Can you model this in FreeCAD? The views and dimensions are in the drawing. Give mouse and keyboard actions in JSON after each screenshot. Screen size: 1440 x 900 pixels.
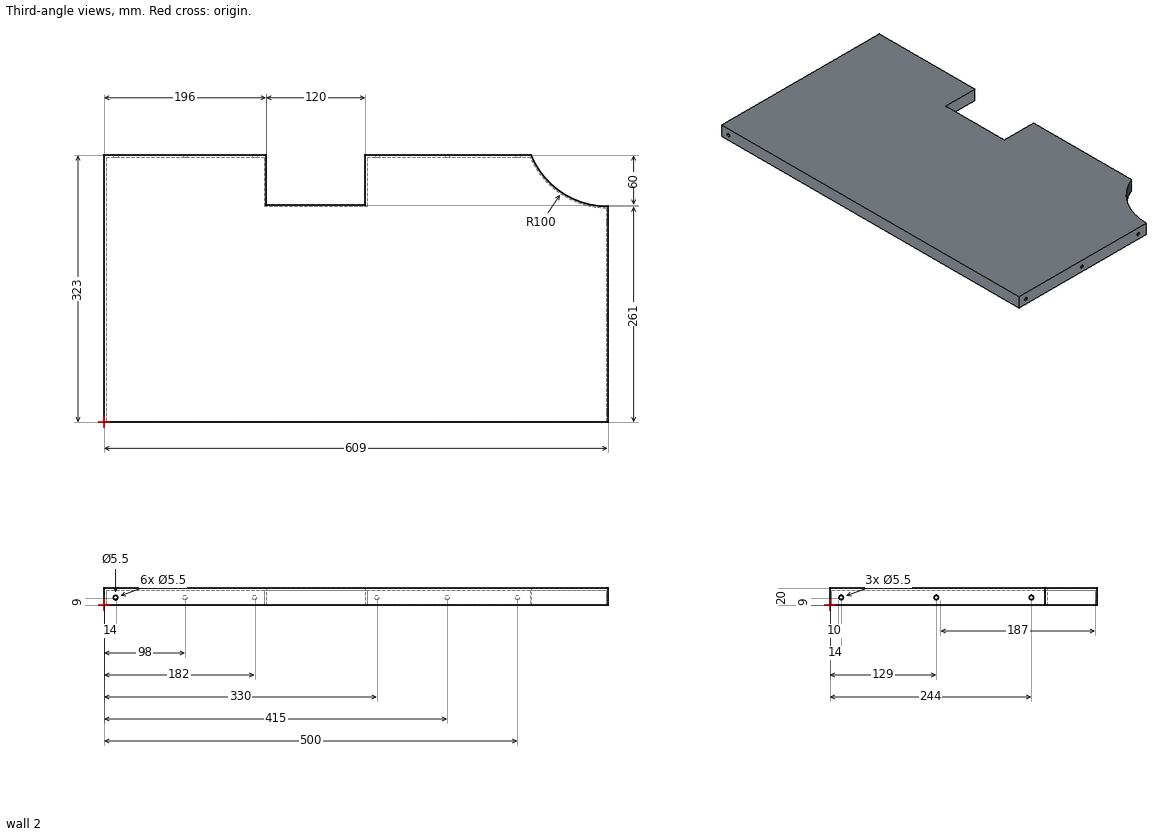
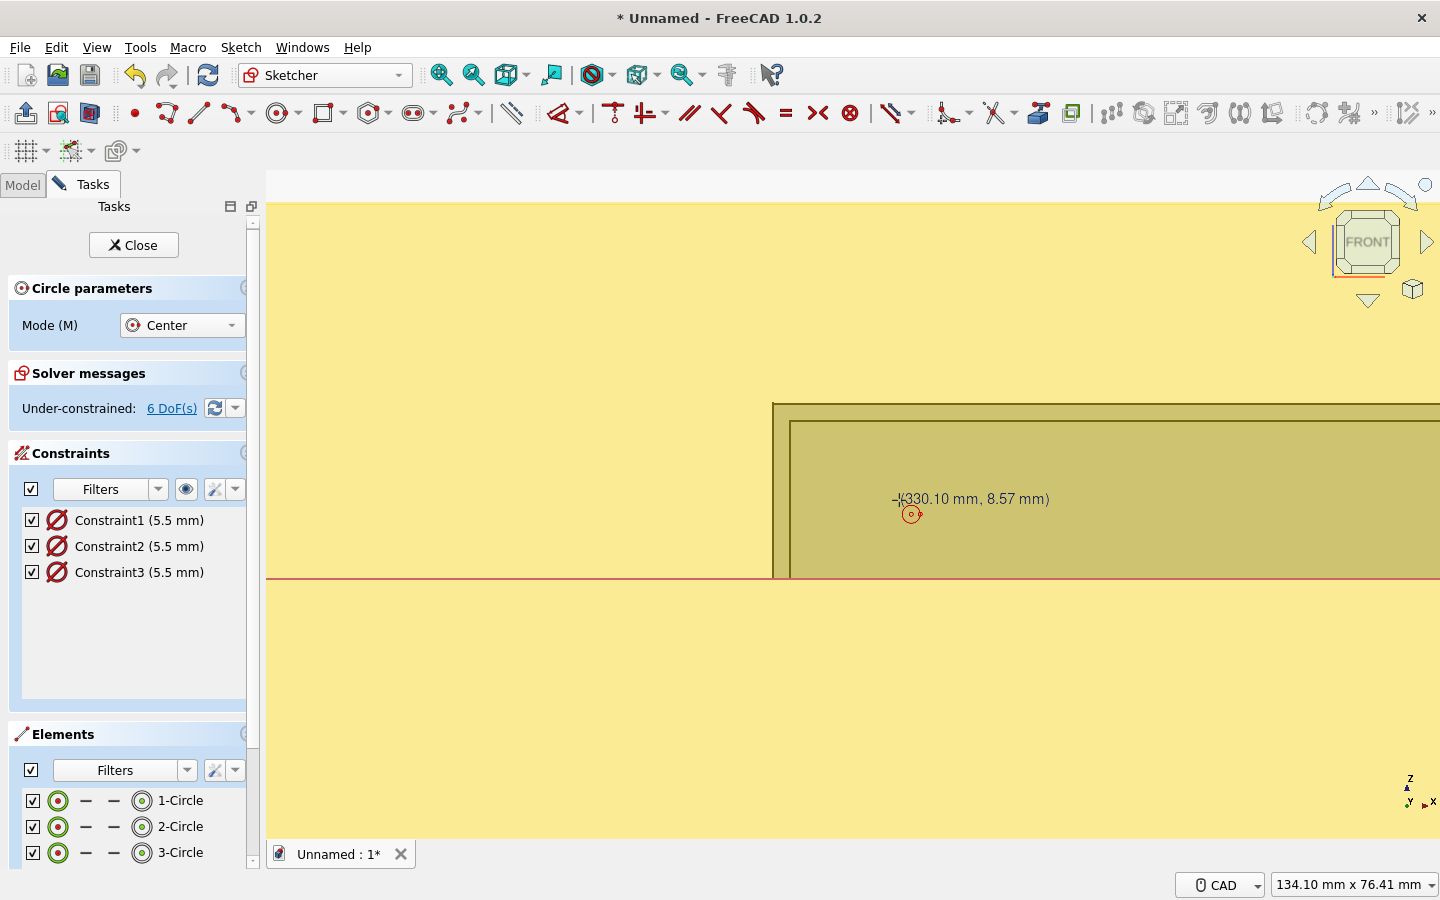
{"action": "scroll", "coordinate": [899, 500], "scroll_direction": "down", "scroll_amount": 9}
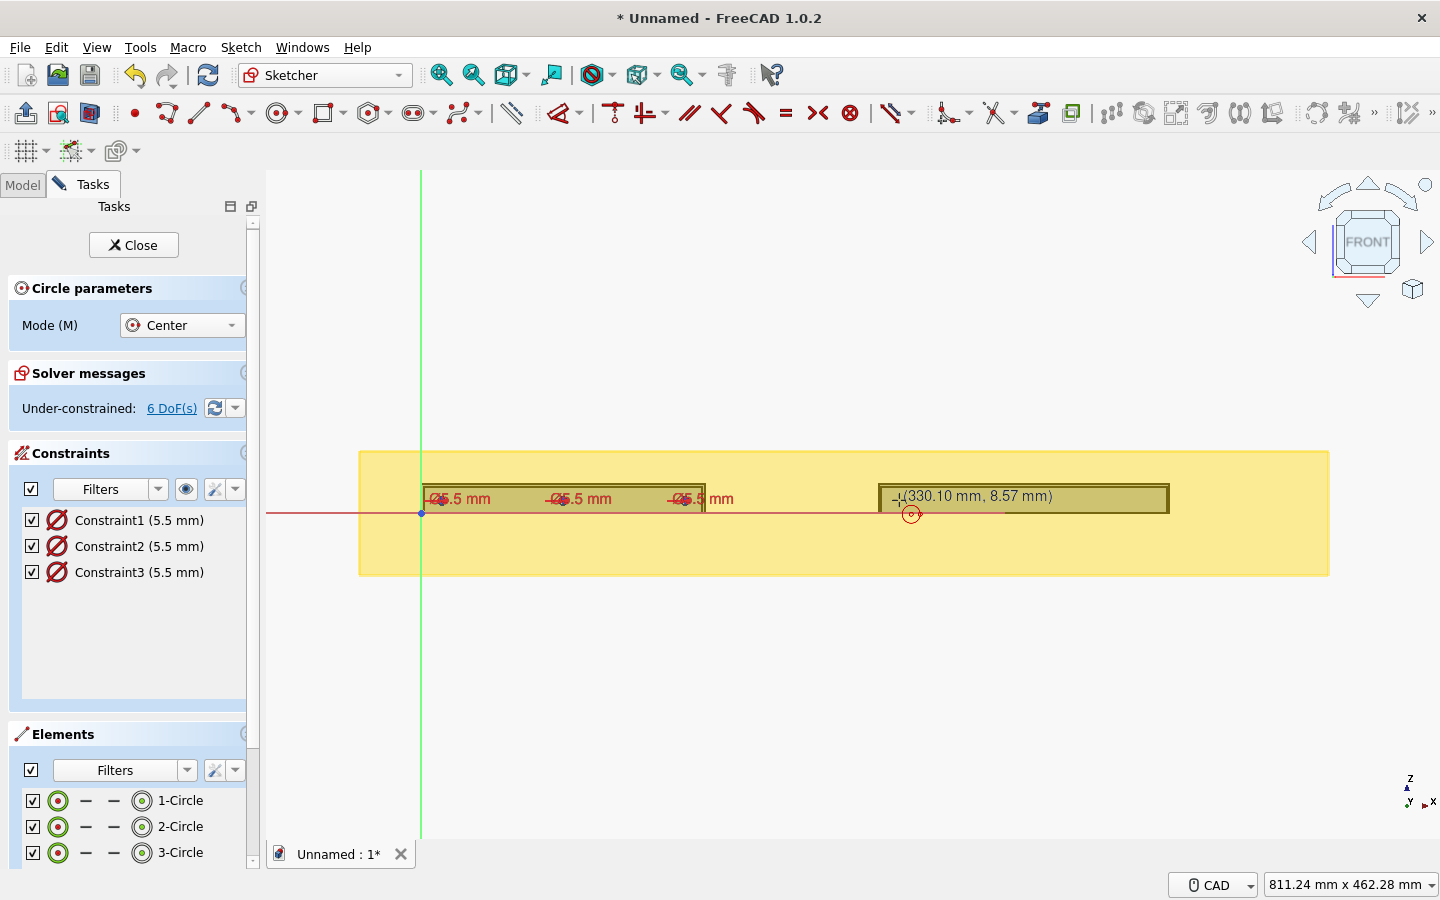
{"action": "left_click", "coordinate": [899, 500]}
{"action": "mouse_move", "coordinate": [902, 498]}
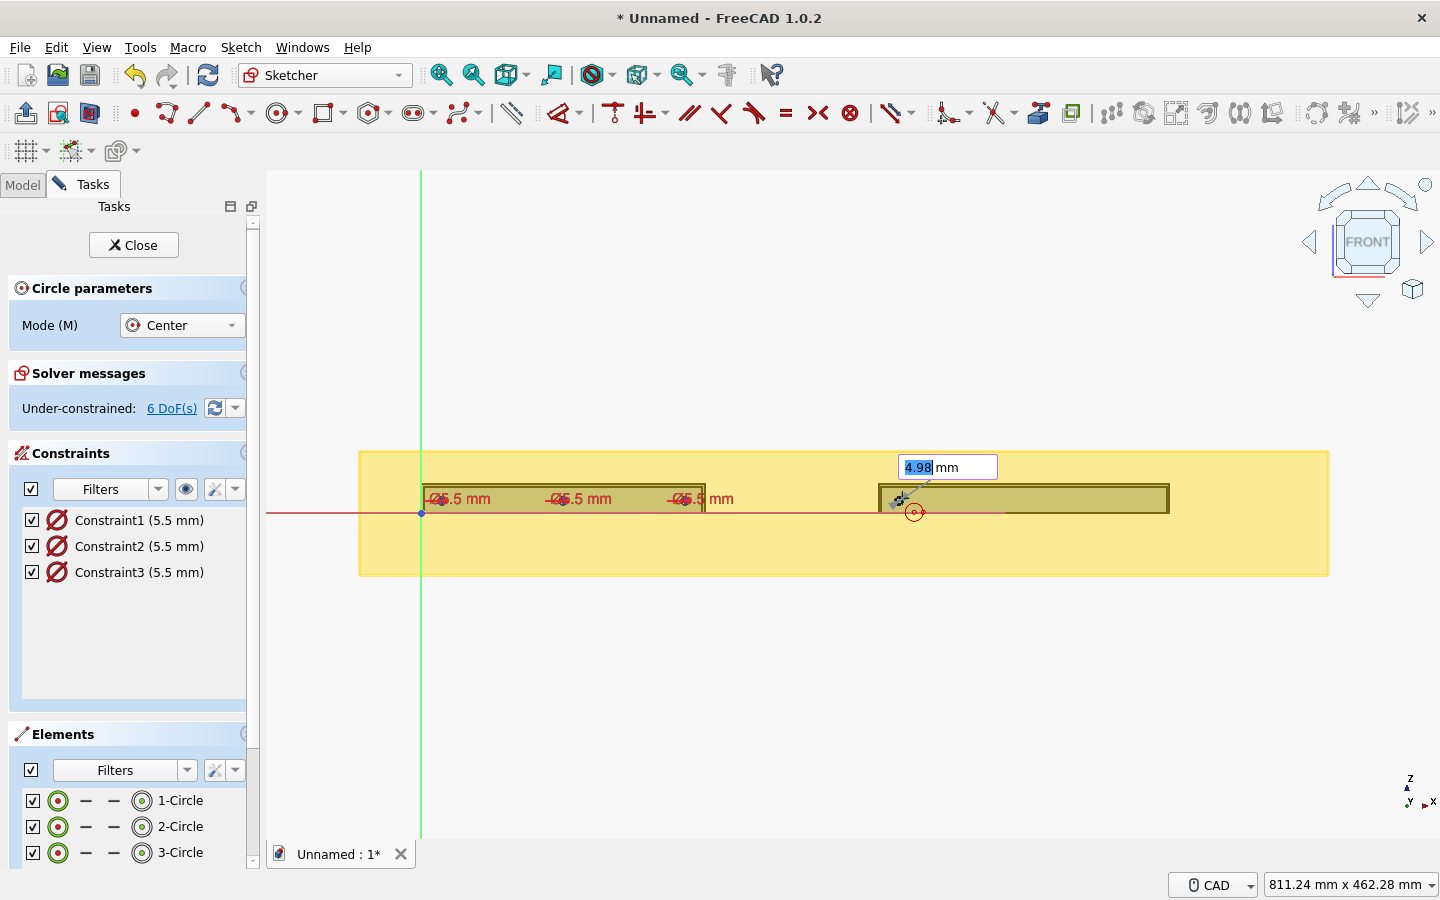
{"action": "type", "text": "5.5"}
{"action": "key", "text": "Return"}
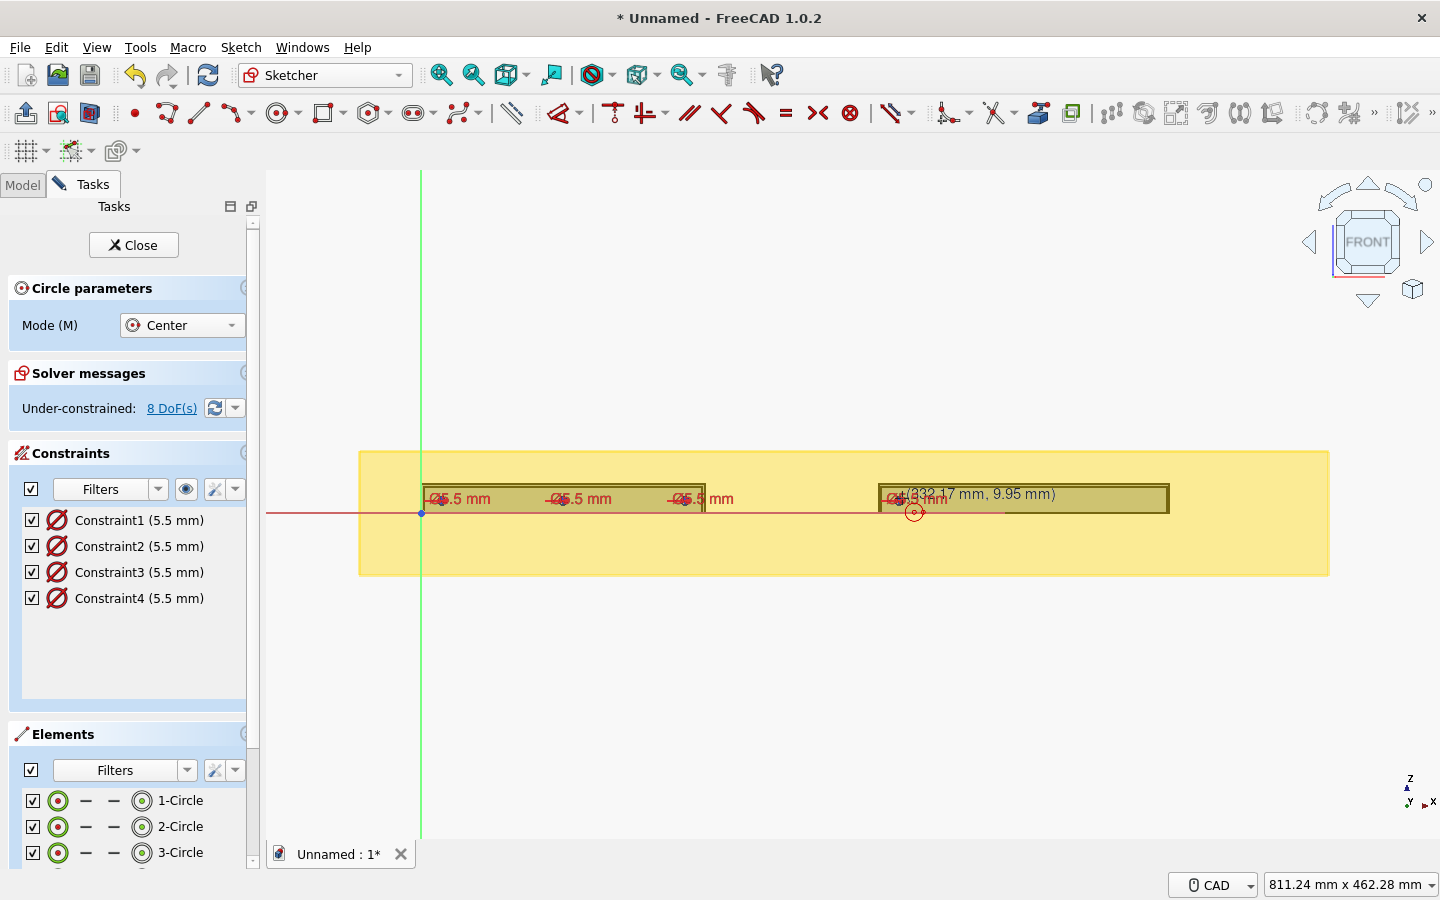
{"action": "scroll", "coordinate": [1145, 500], "scroll_direction": "up", "scroll_amount": 9}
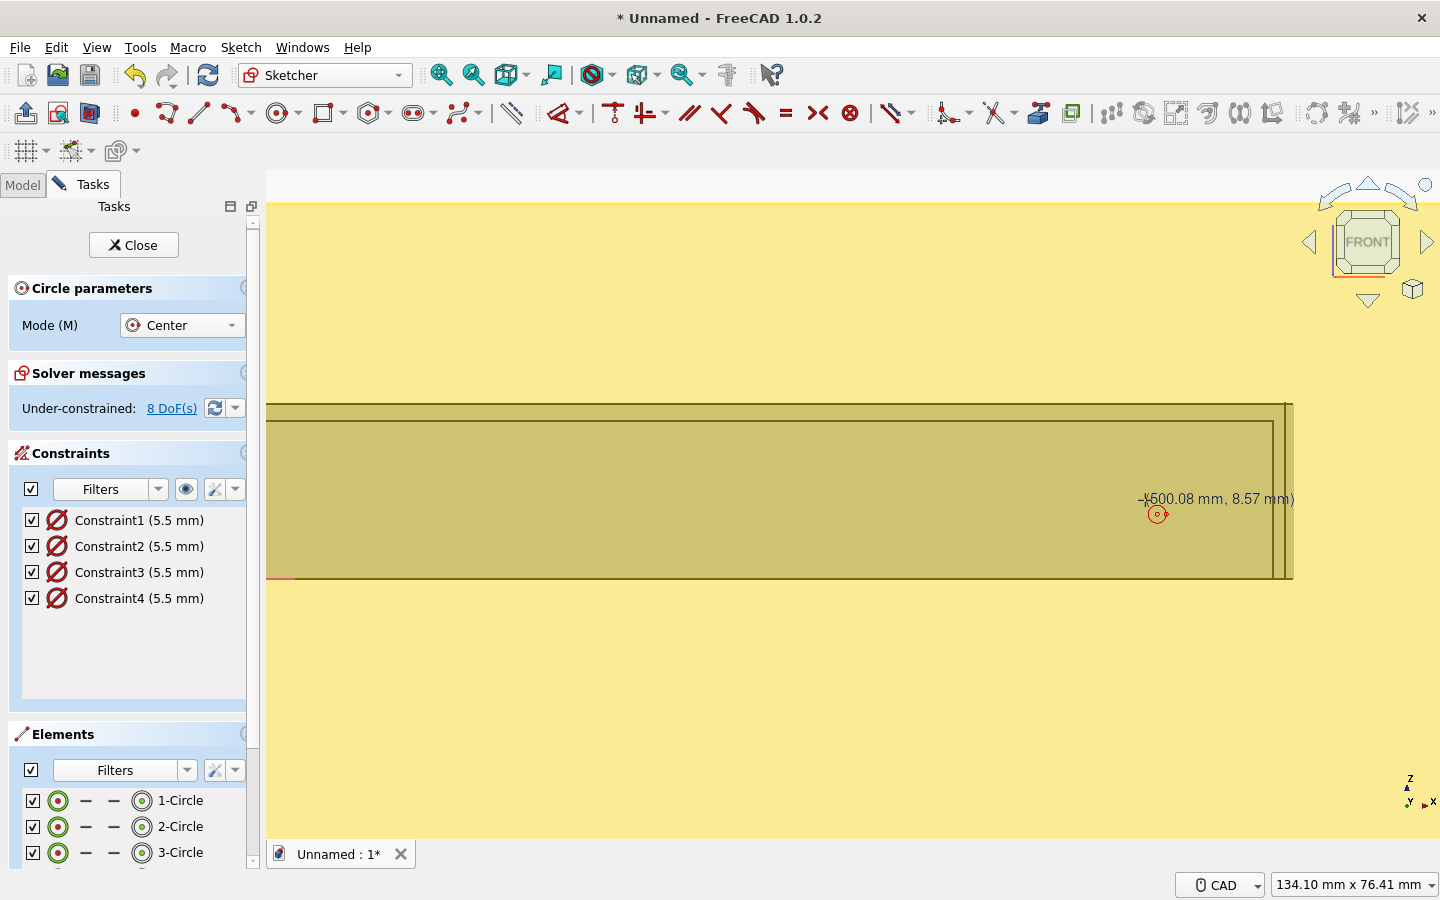
{"action": "scroll", "coordinate": [1145, 500], "scroll_direction": "down", "scroll_amount": 9}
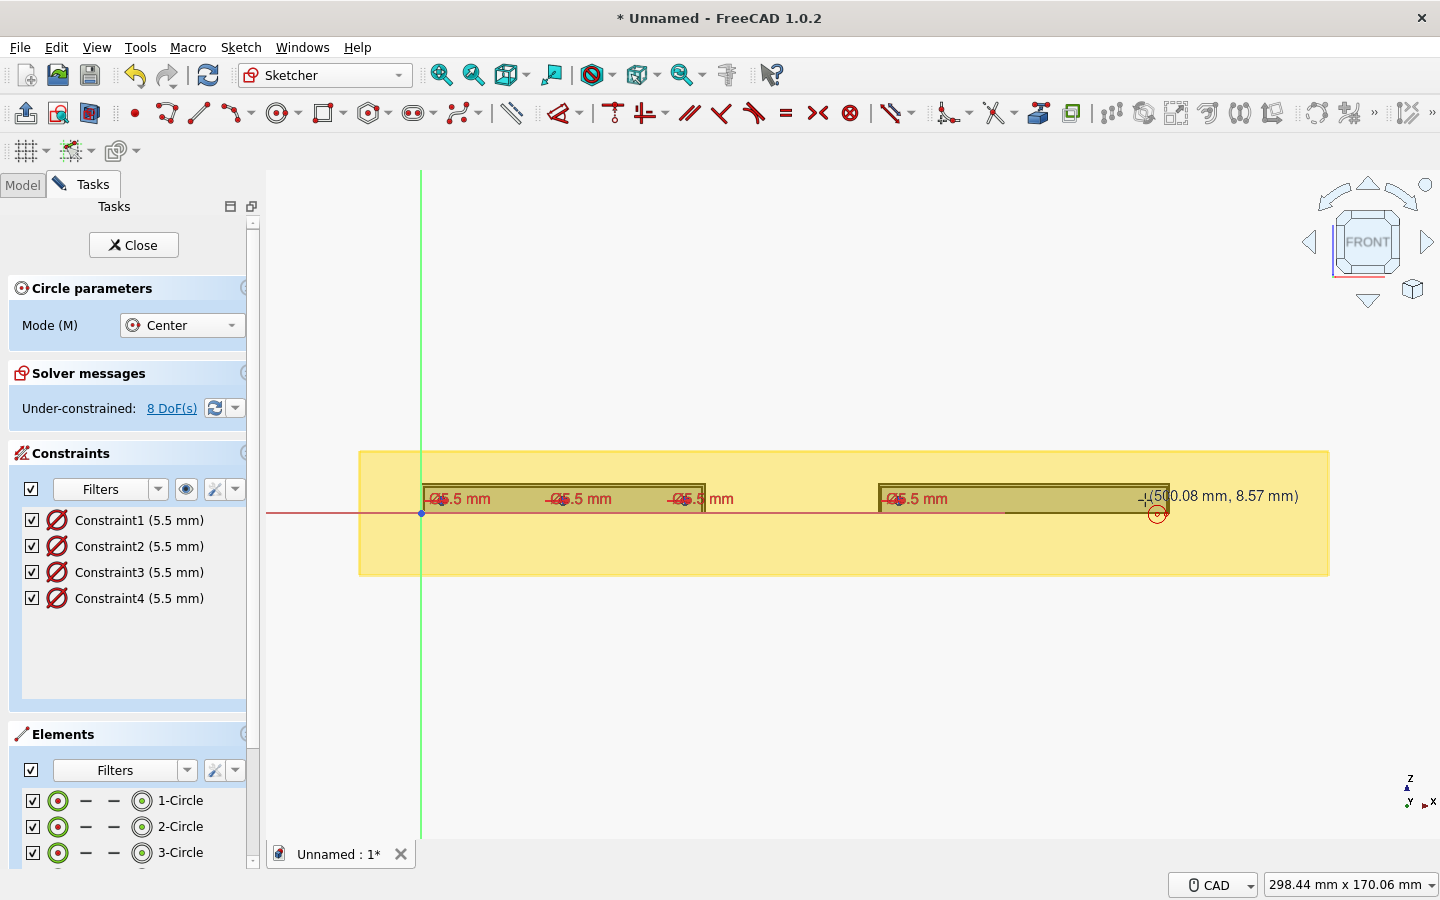
{"action": "left_click", "coordinate": [1145, 500]}
{"action": "mouse_move", "coordinate": [1148, 498]}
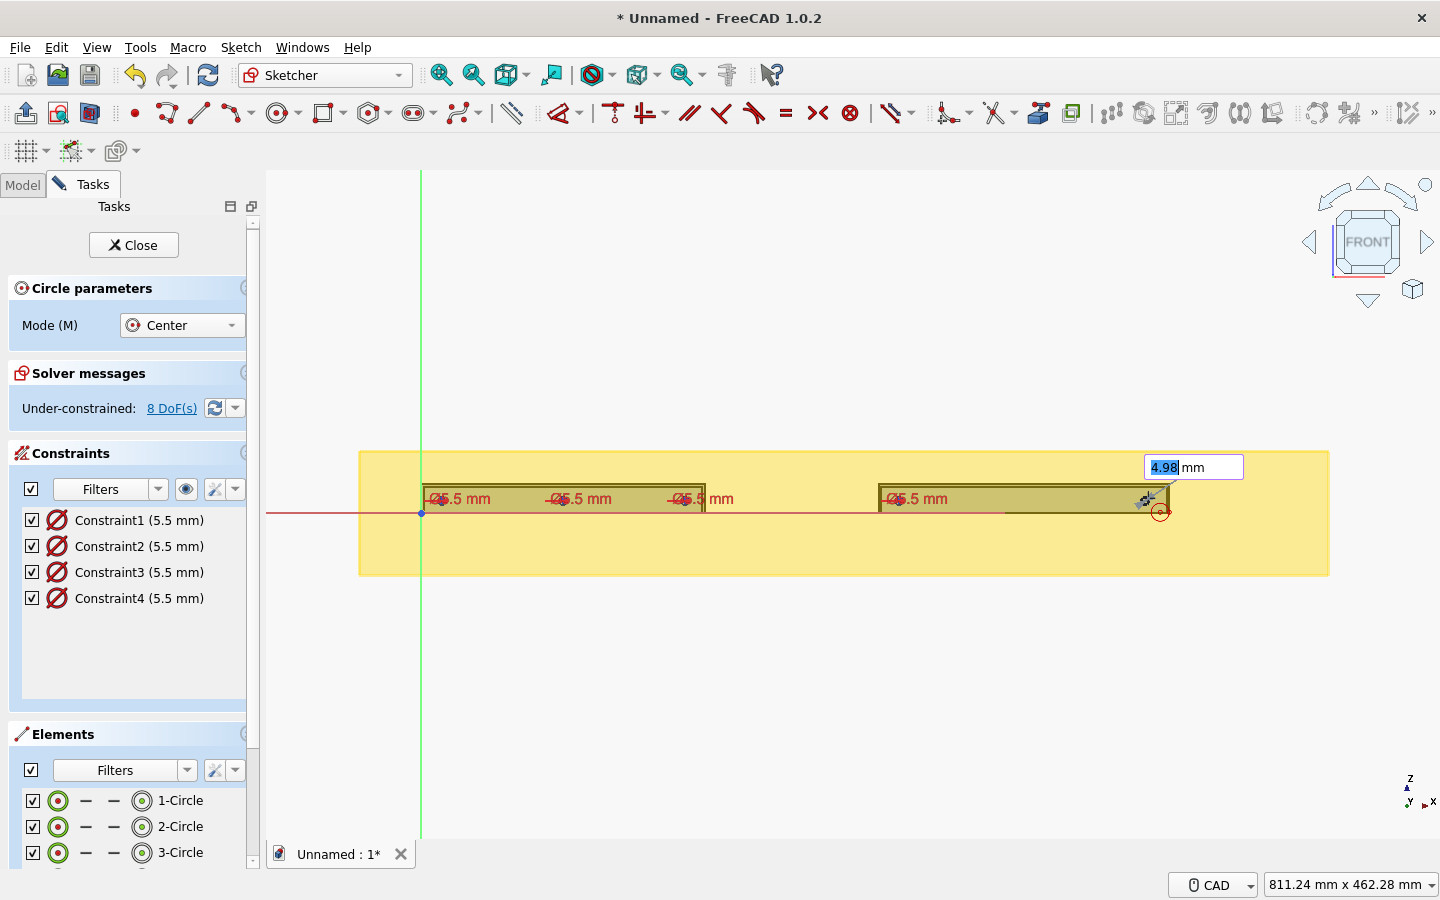
{"action": "type", "text": "5.5"}
{"action": "key", "text": "Return"}